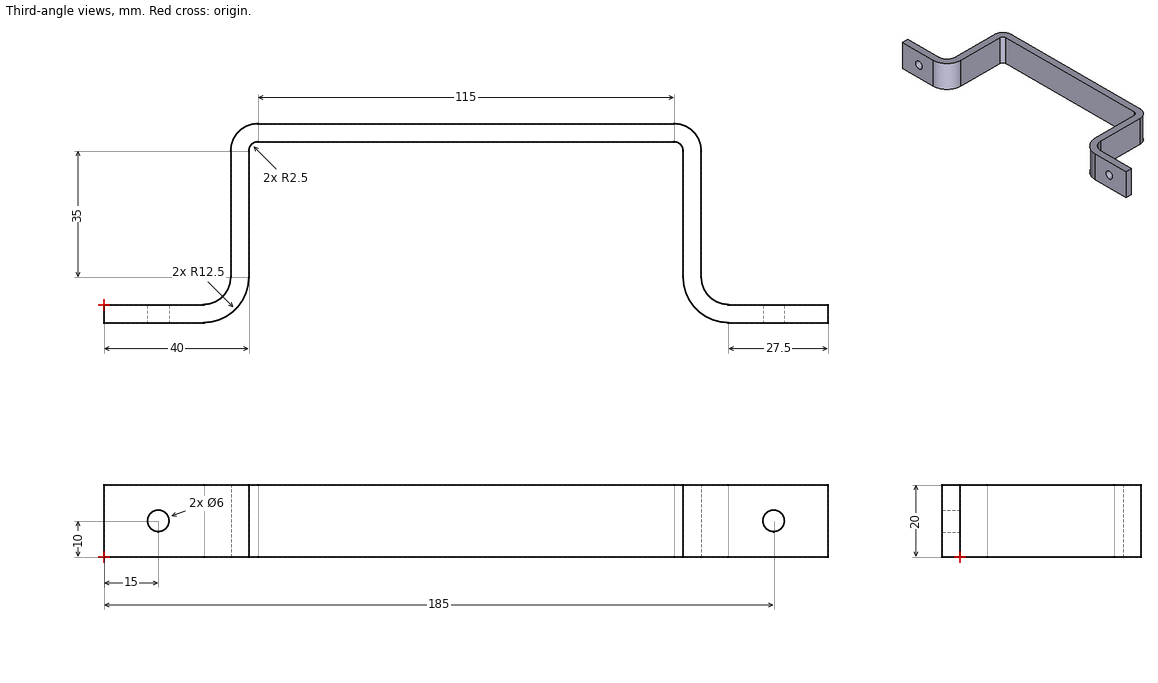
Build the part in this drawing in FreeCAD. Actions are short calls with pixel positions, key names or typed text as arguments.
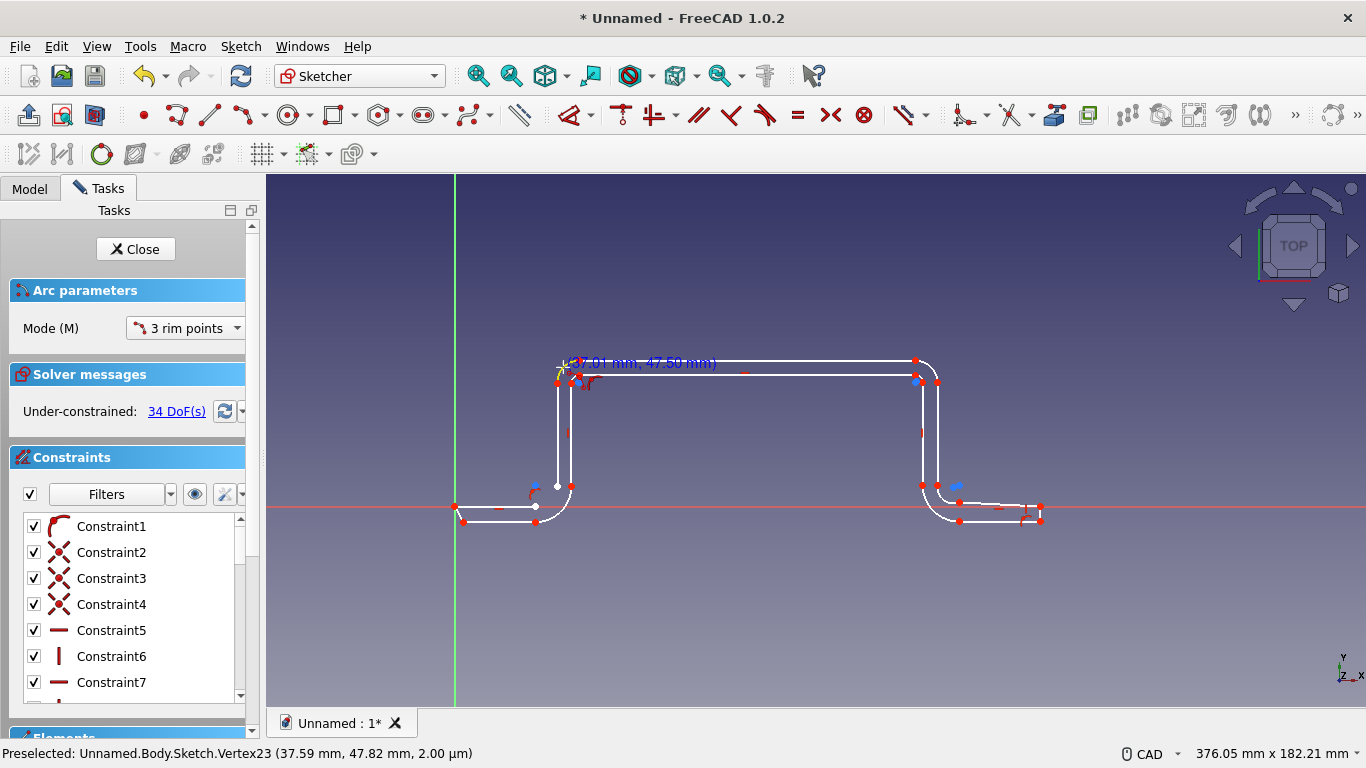
click(558, 486)
click(535, 507)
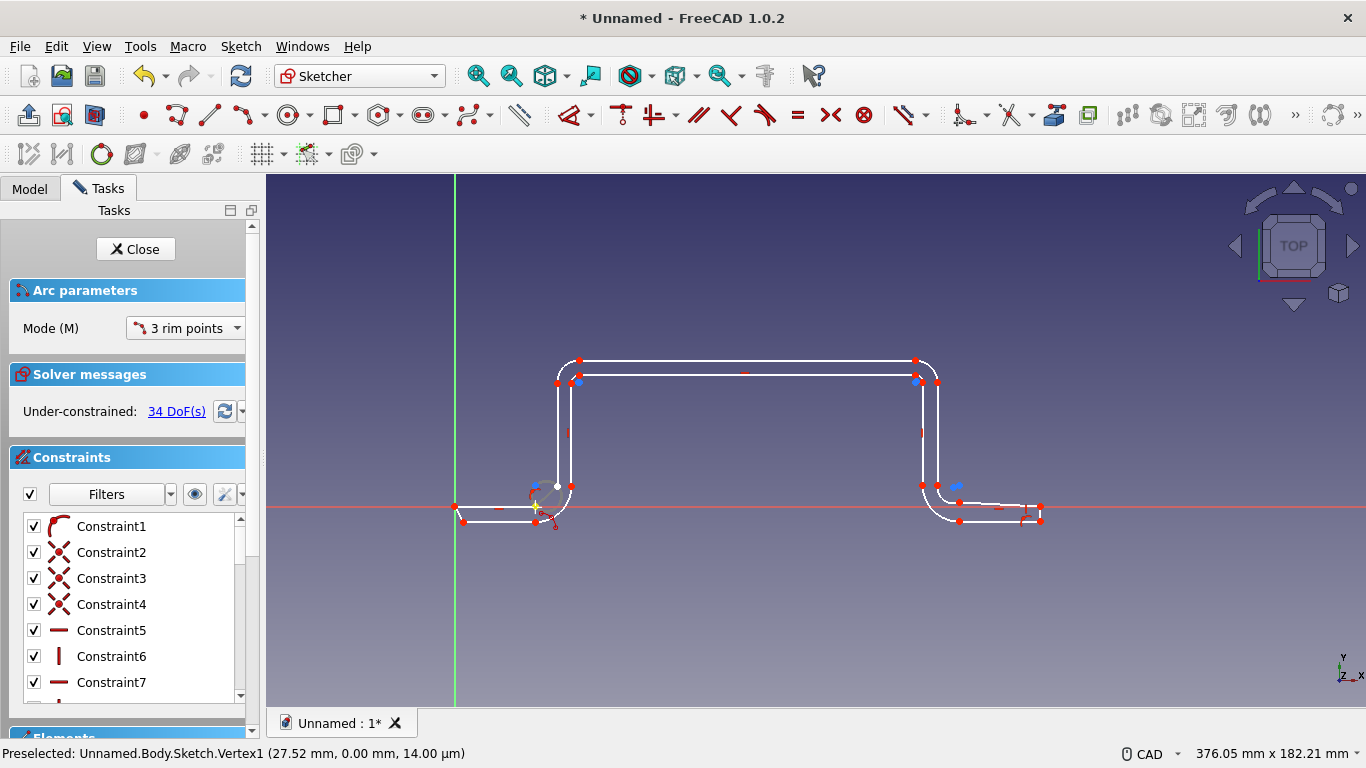
scroll(551, 500, up, 5)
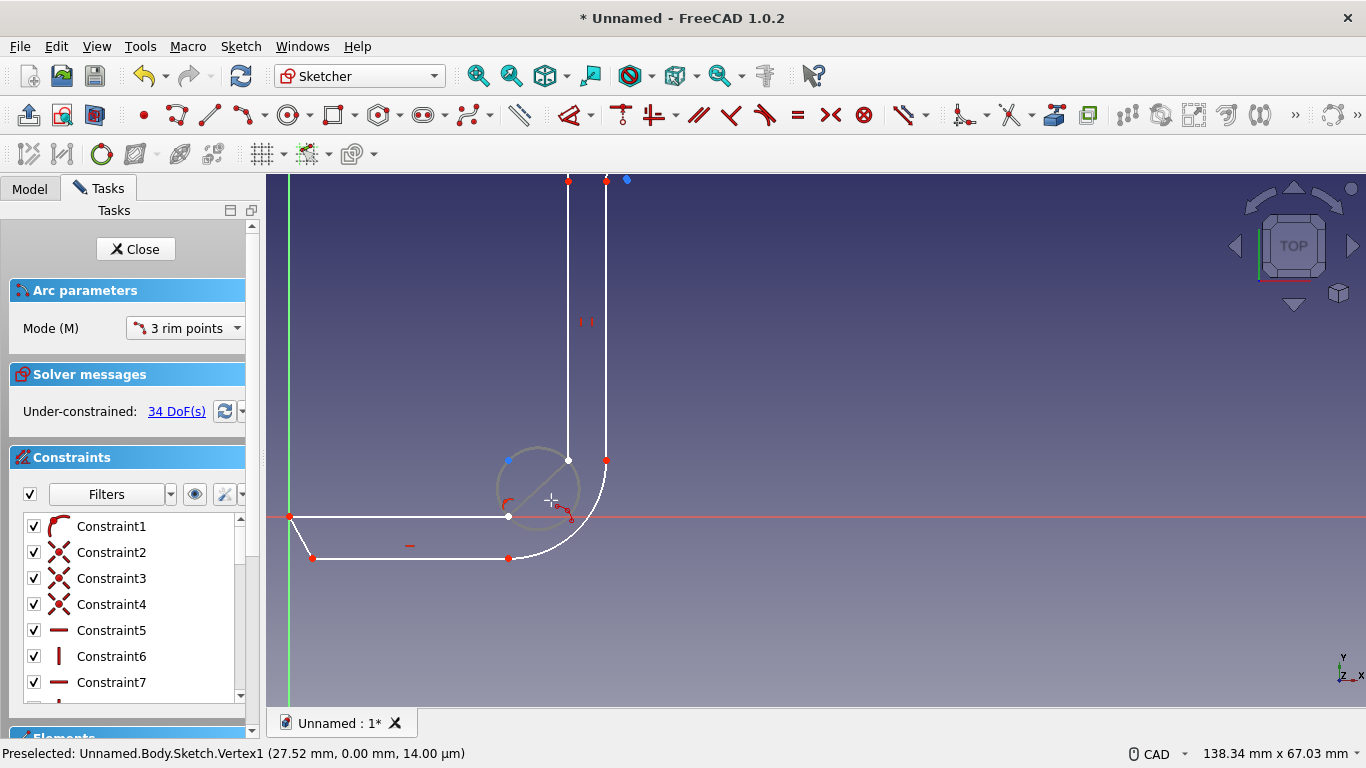
click(550, 499)
key(Escape)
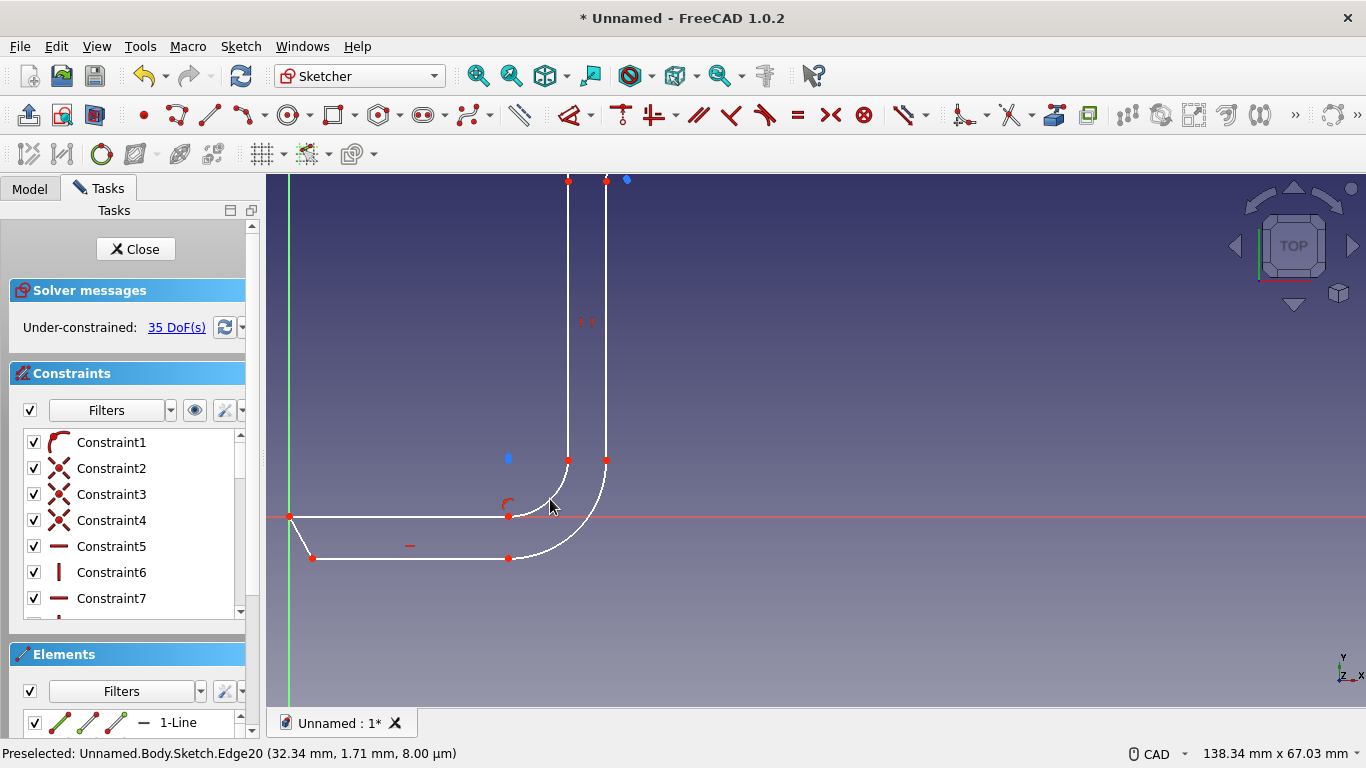
click(443, 517)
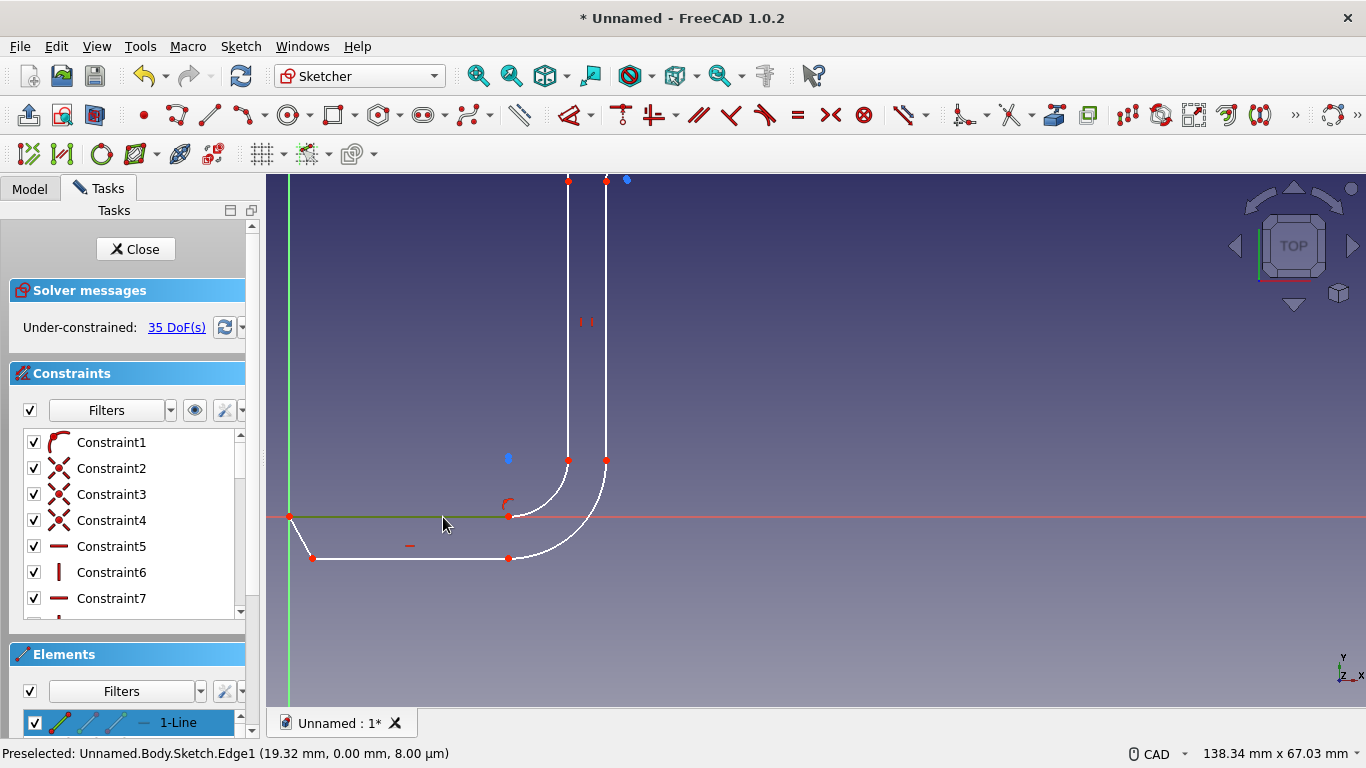
click(560, 487)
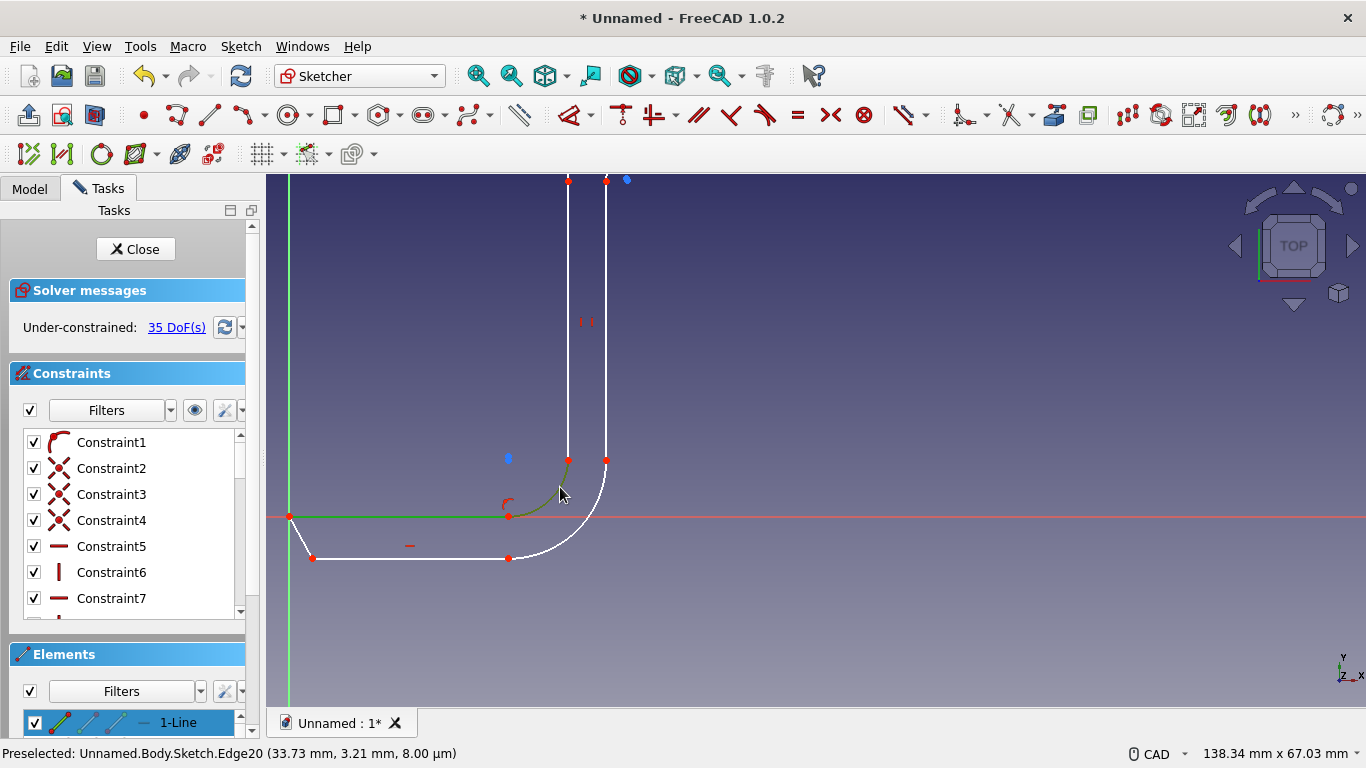
click(765, 116)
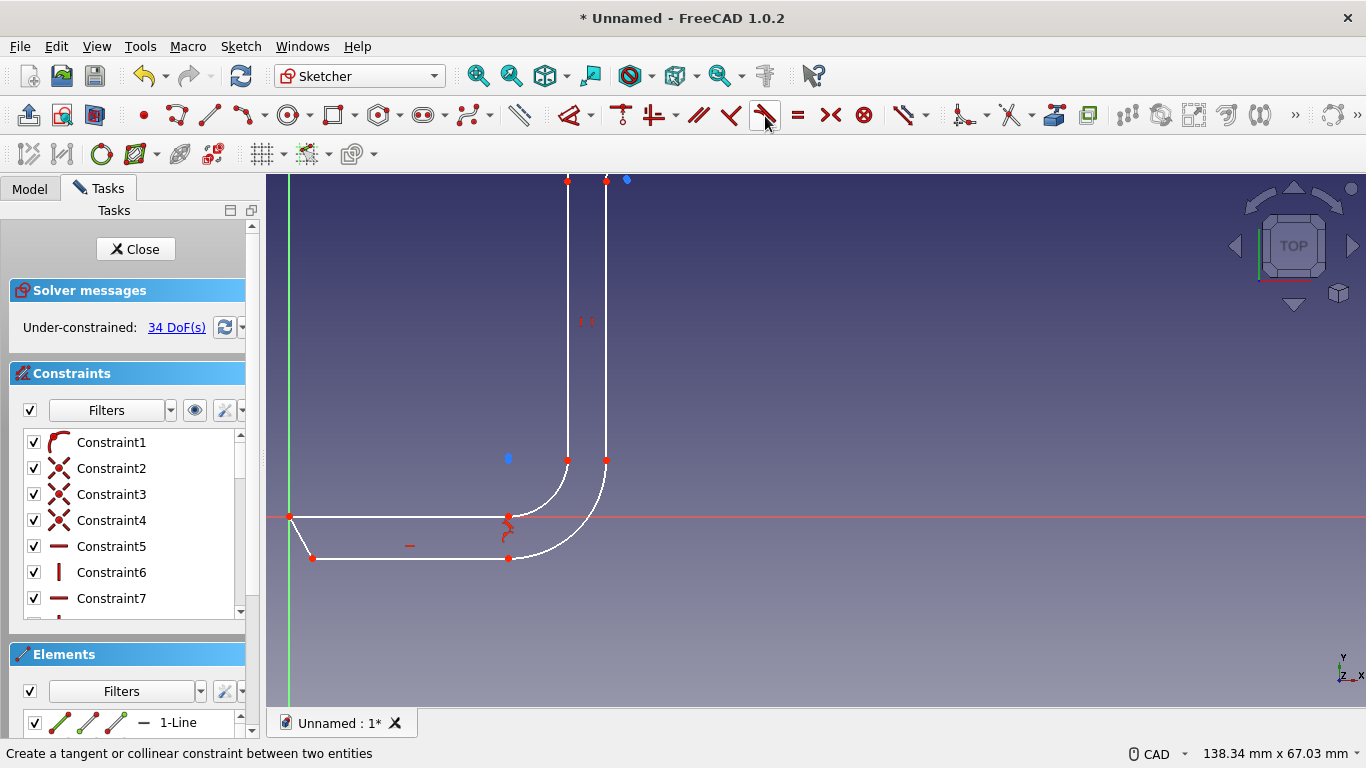
click(371, 559)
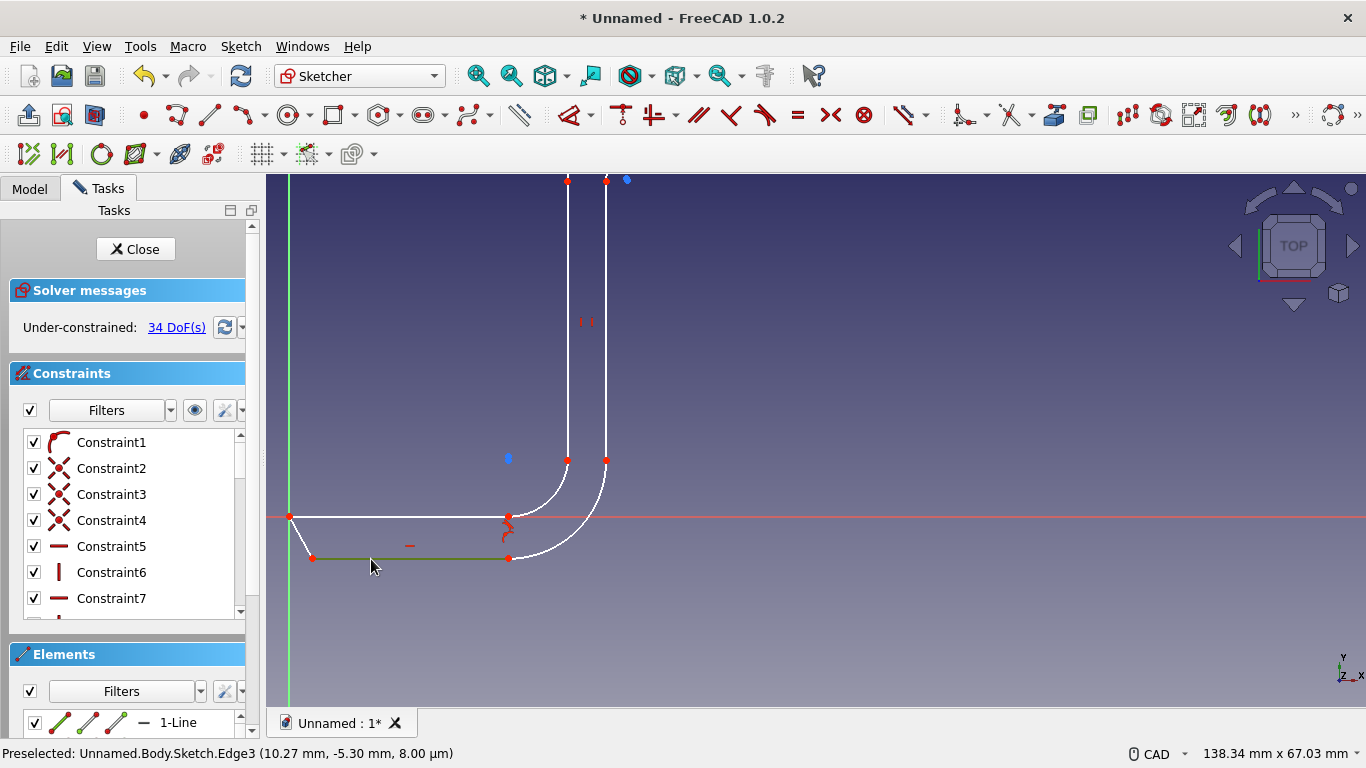
click(553, 548)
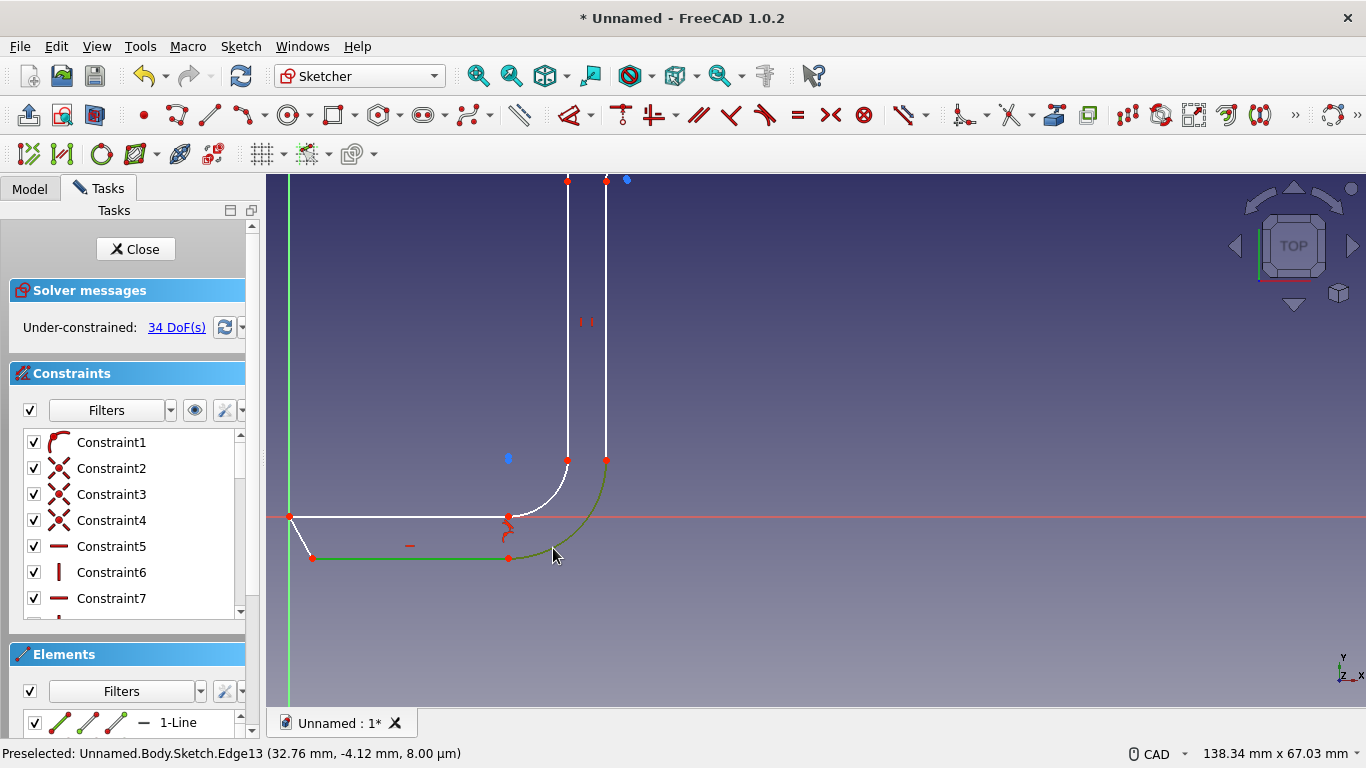
key(t)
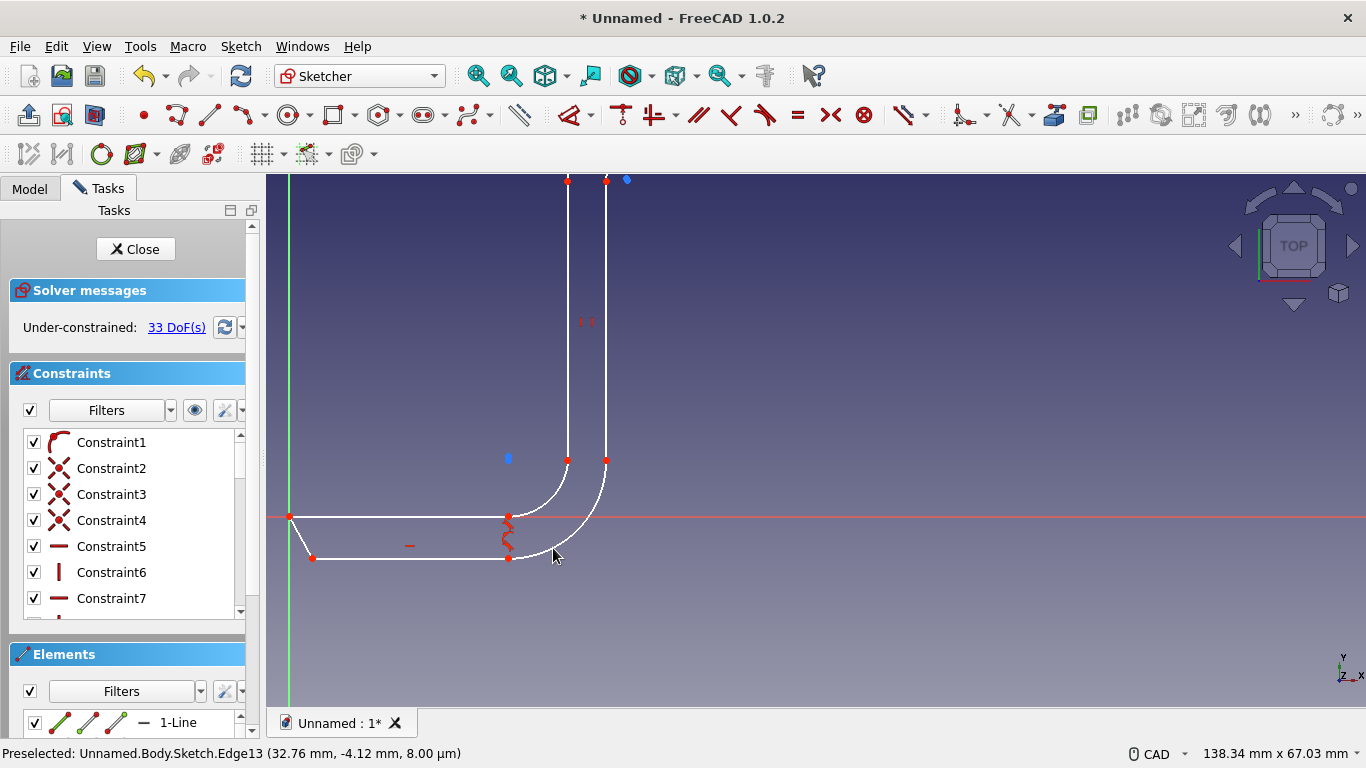
click(606, 377)